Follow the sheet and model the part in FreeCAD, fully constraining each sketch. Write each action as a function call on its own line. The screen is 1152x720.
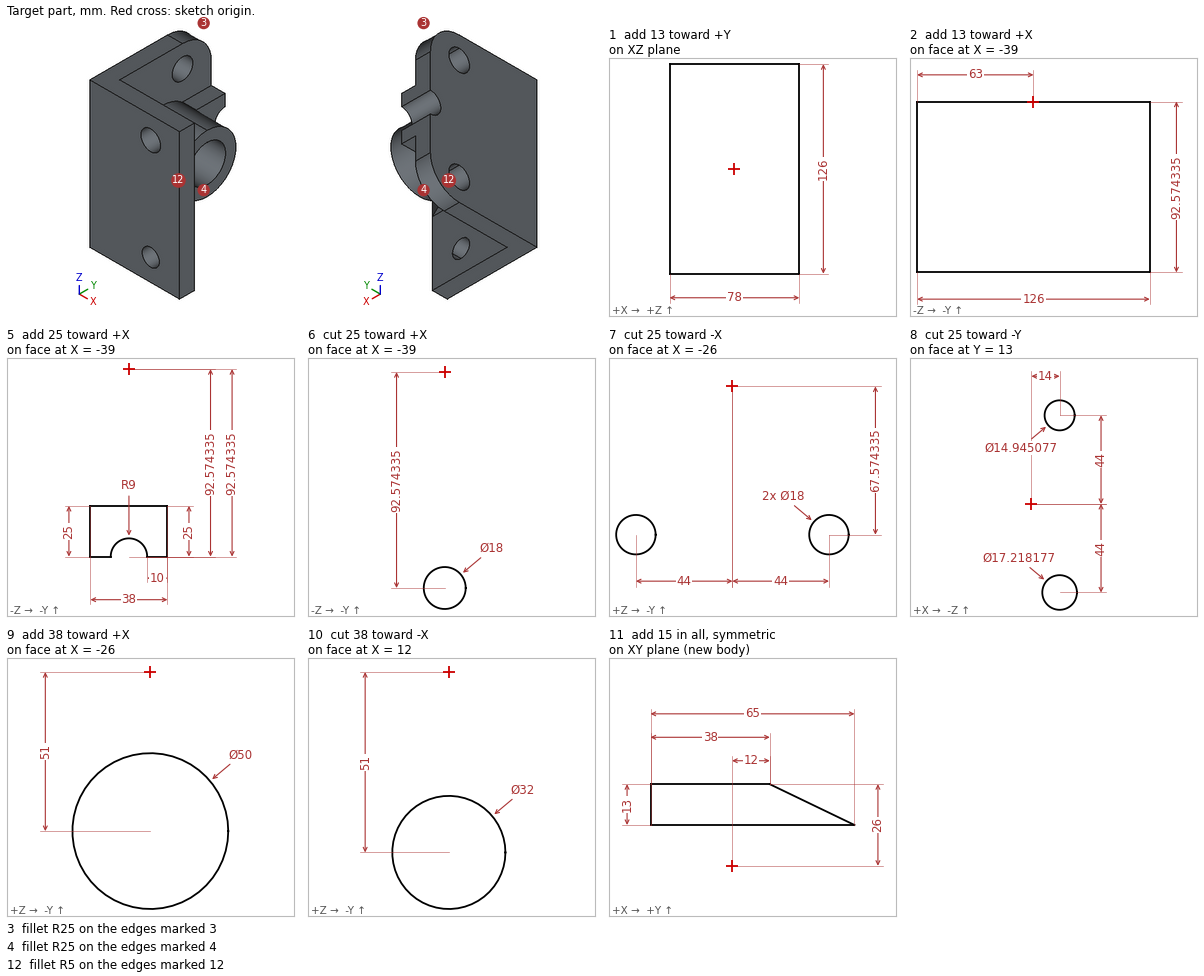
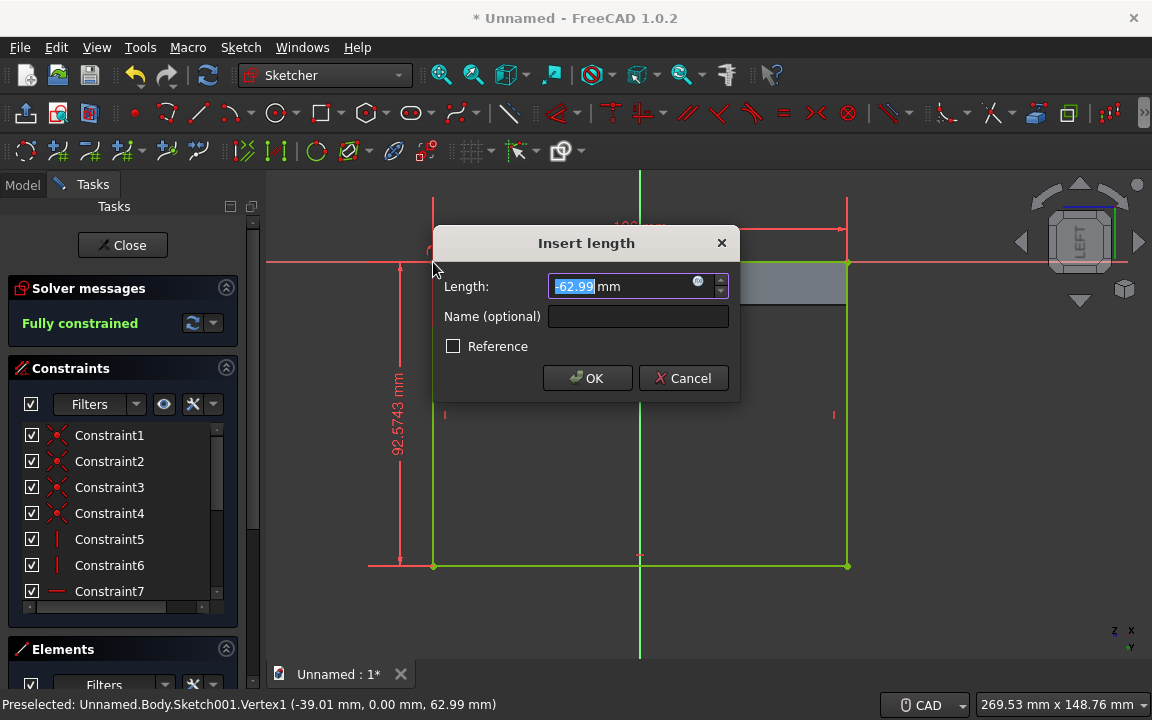
text(-63)
key(Return)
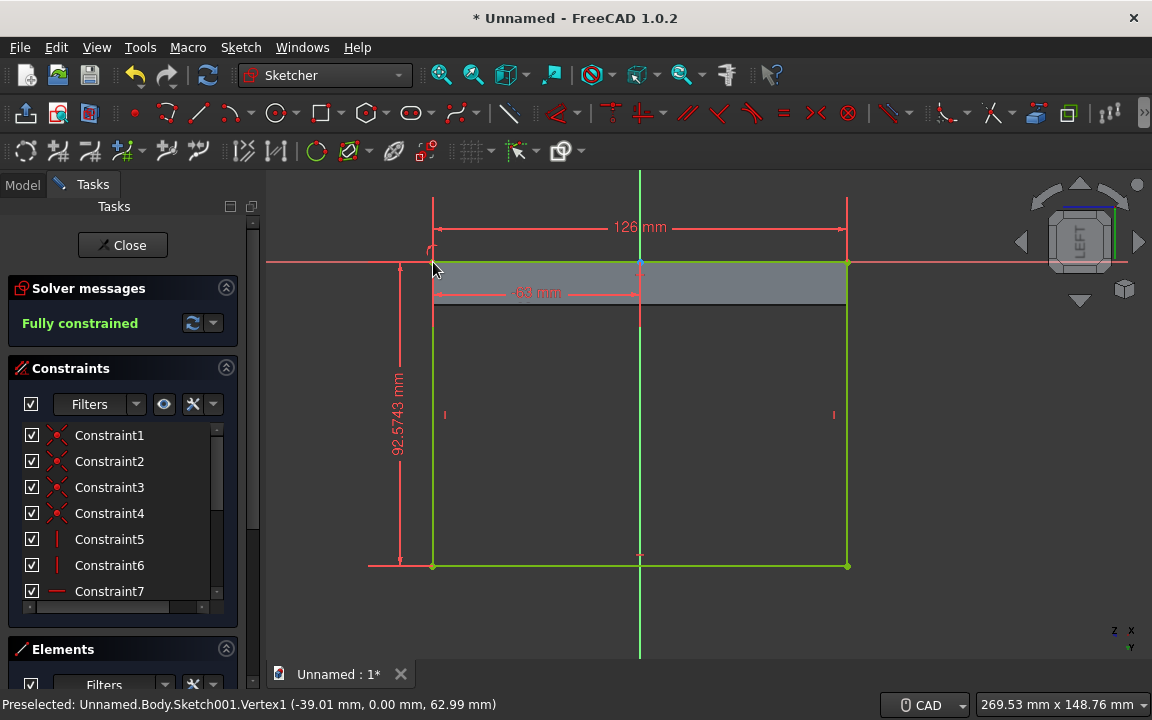
click(123, 245)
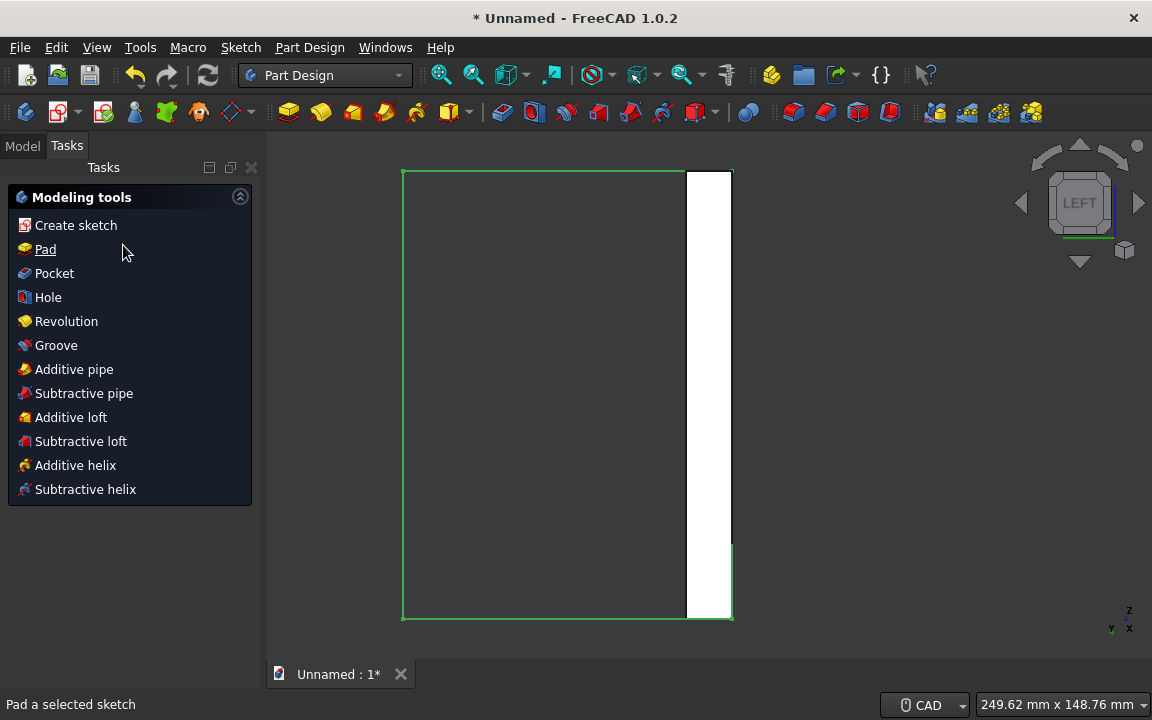
click(290, 112)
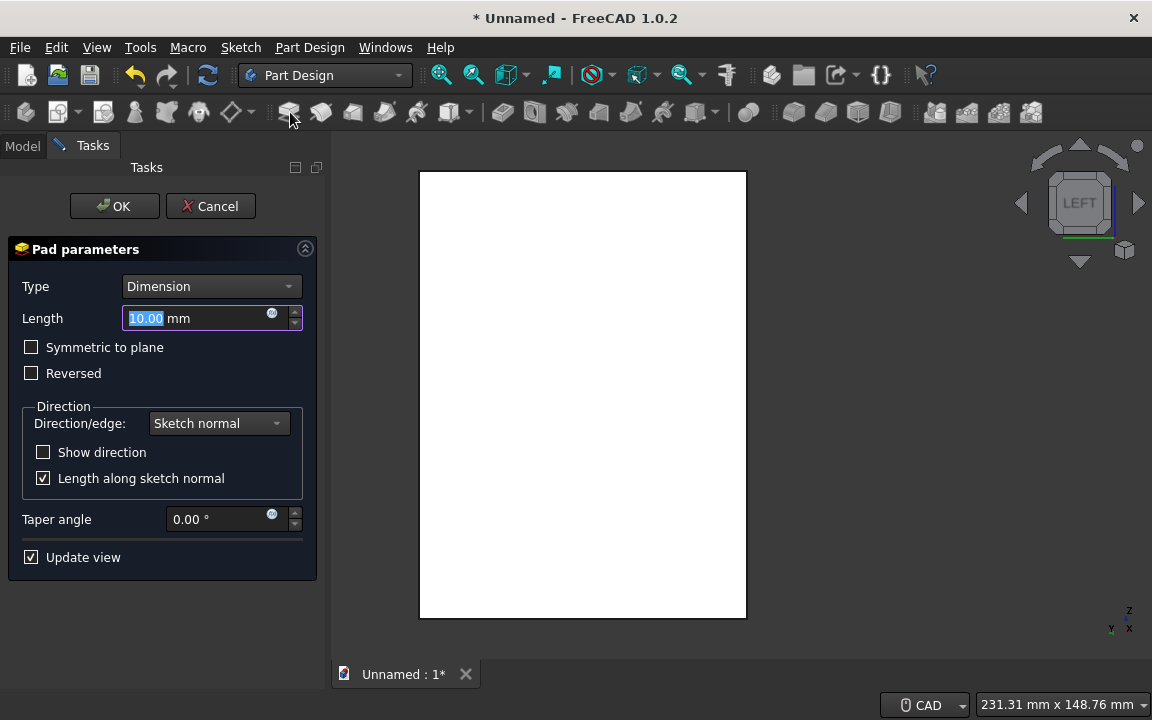
text(13)
key(Tab)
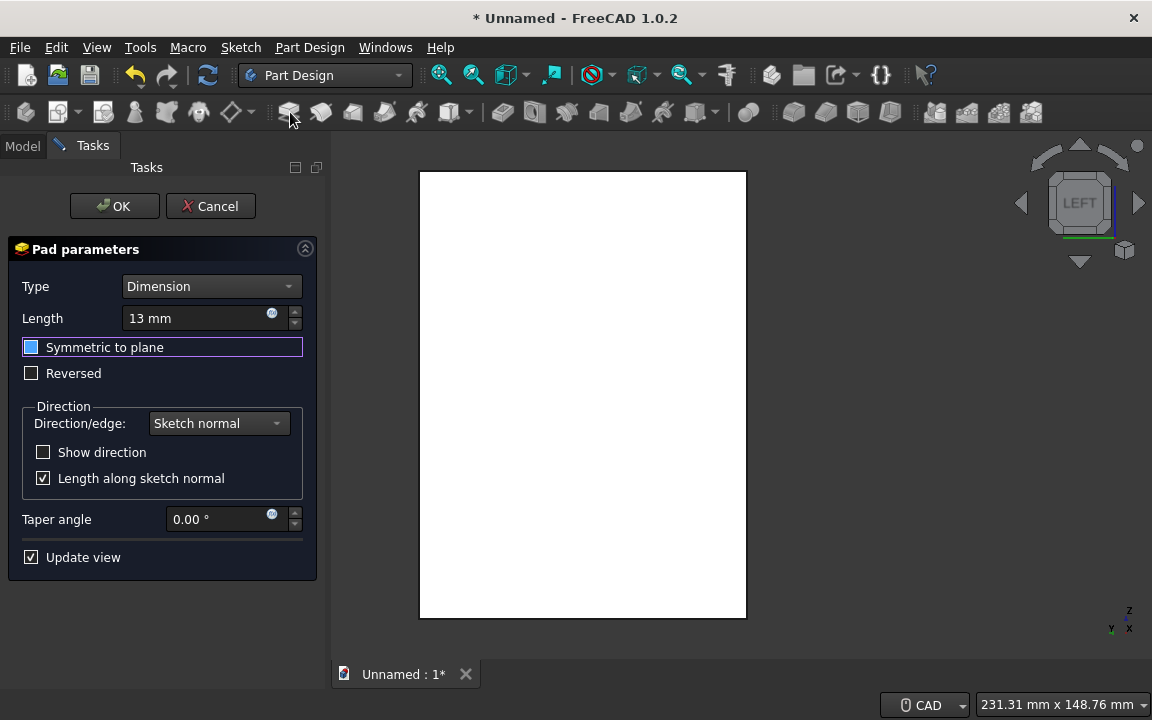
click(30, 373)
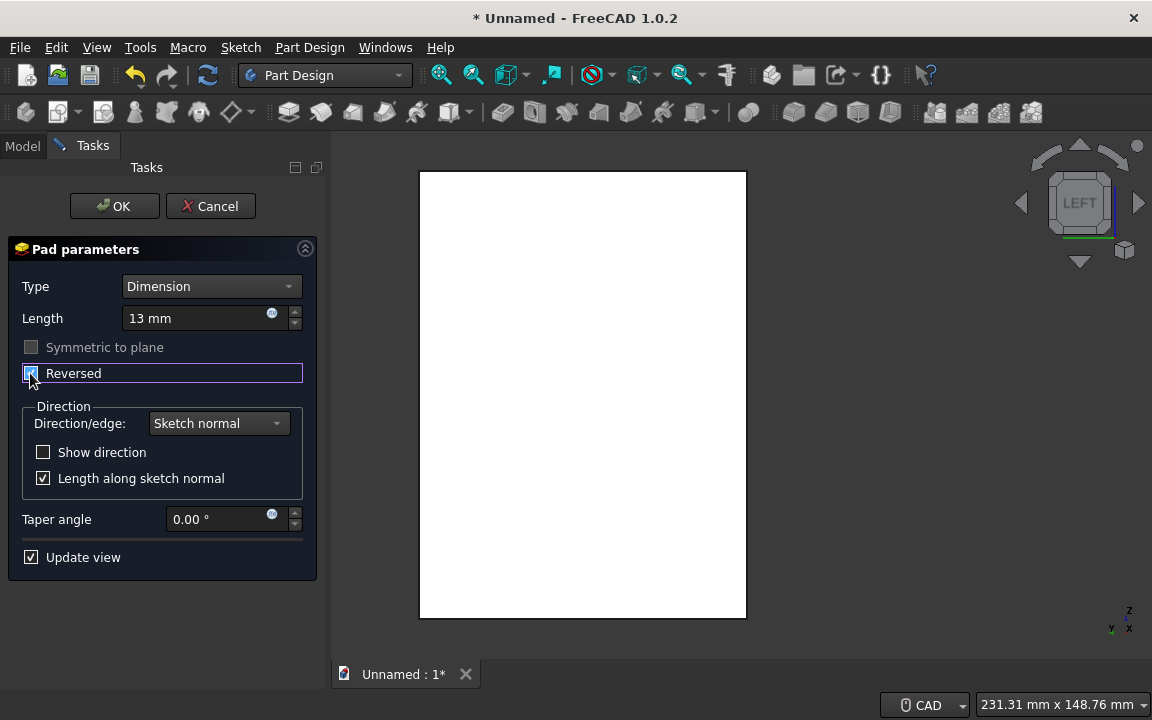
click(115, 206)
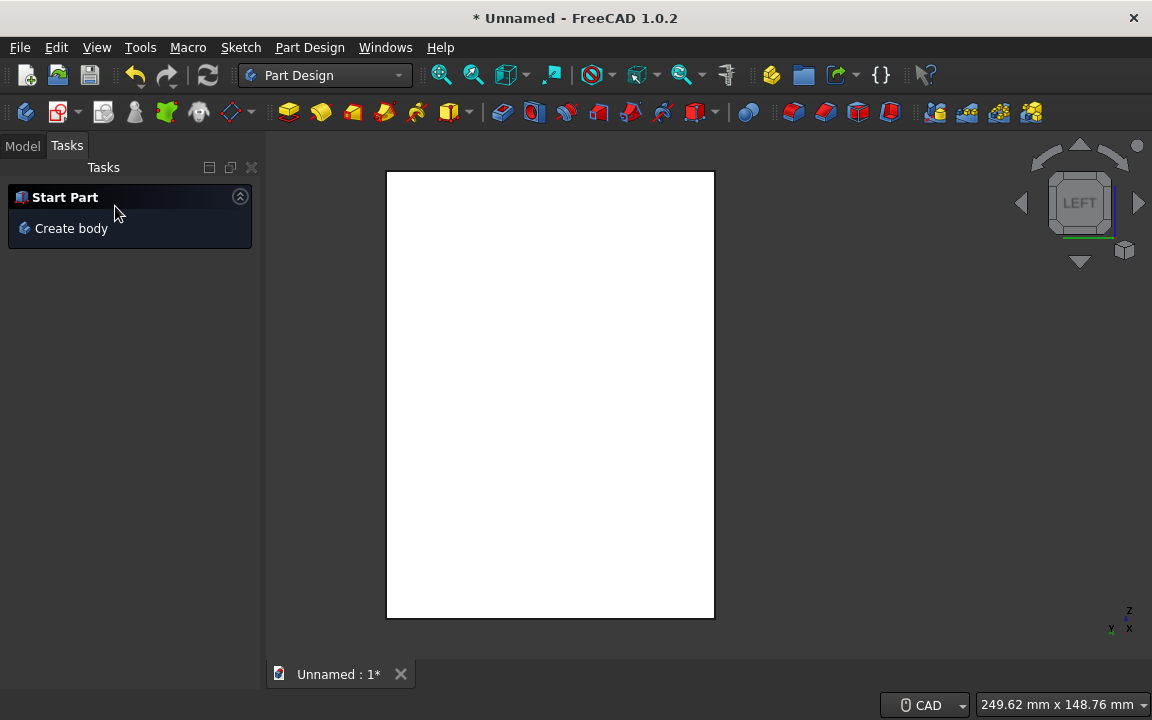
key(0)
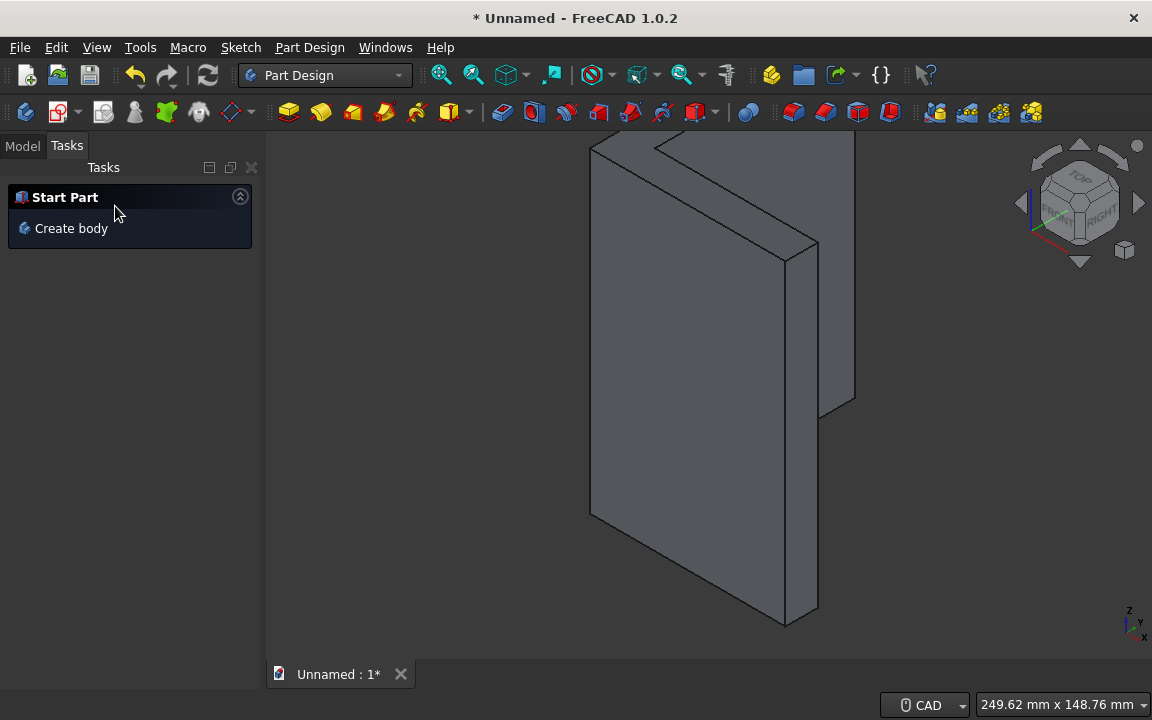
key(v)
key(f)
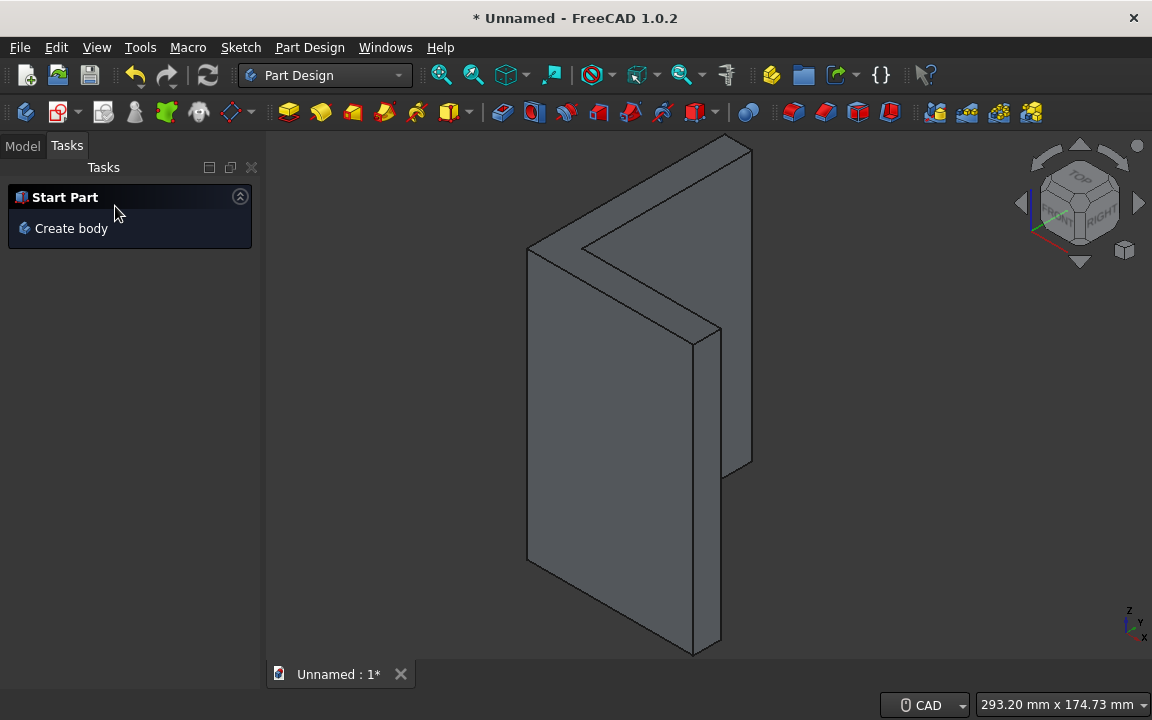
key(2)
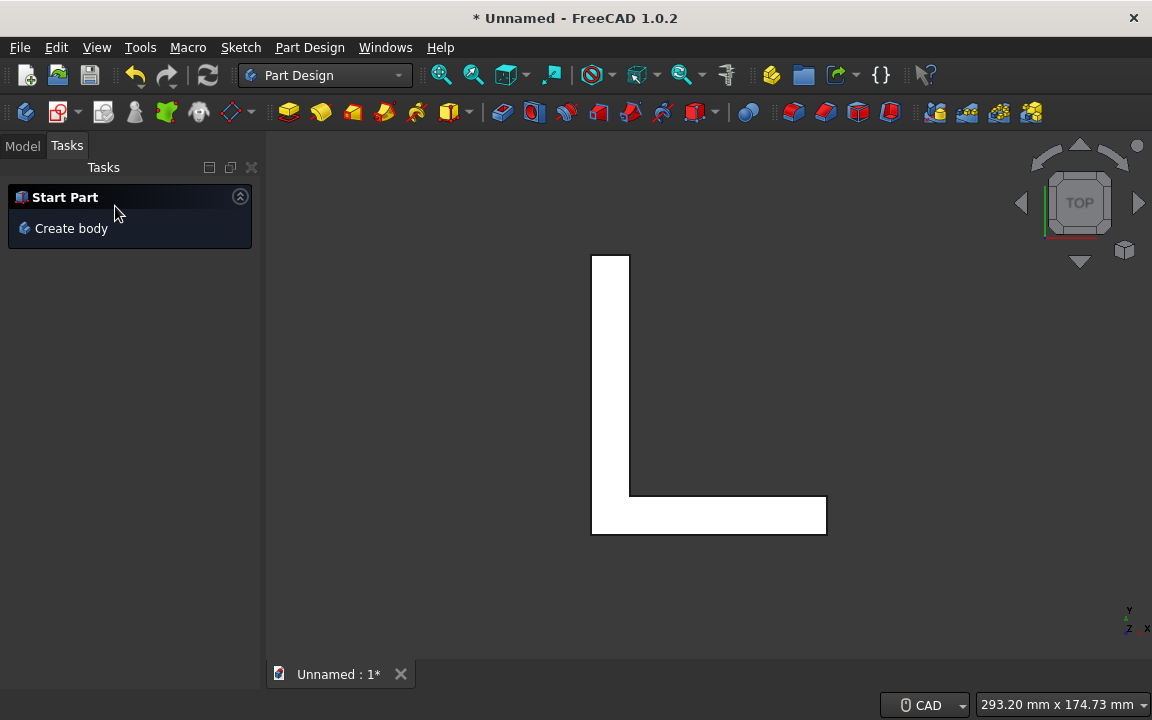
click(611, 254)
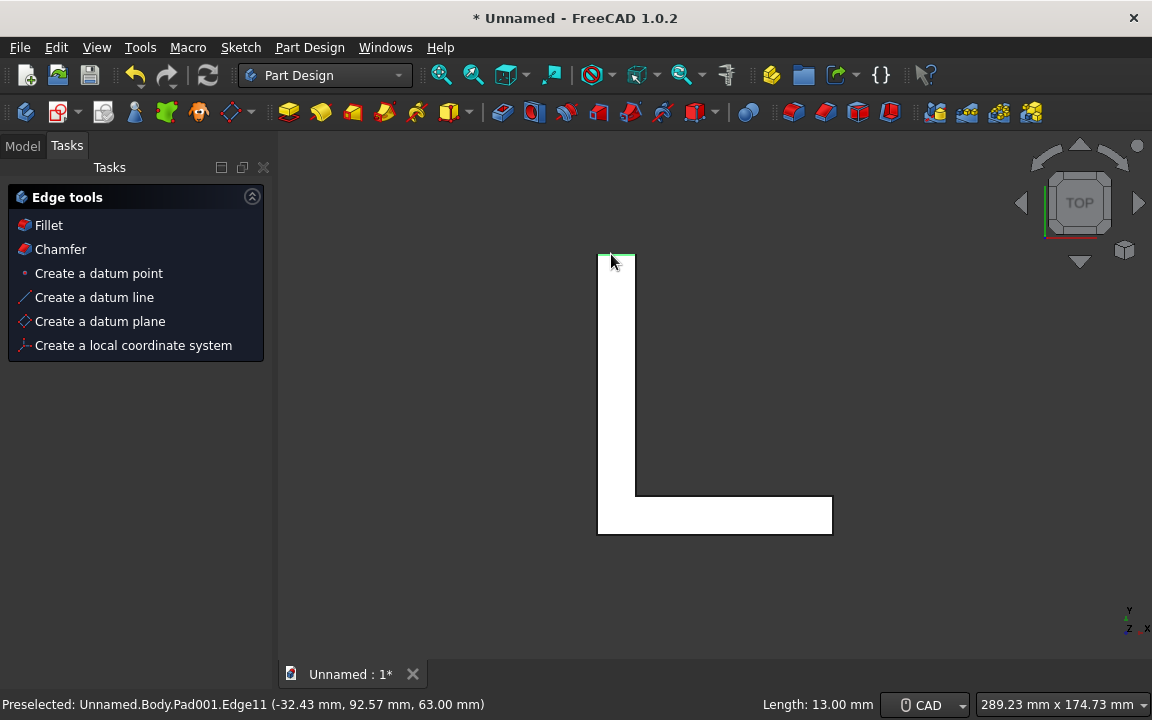
click(794, 112)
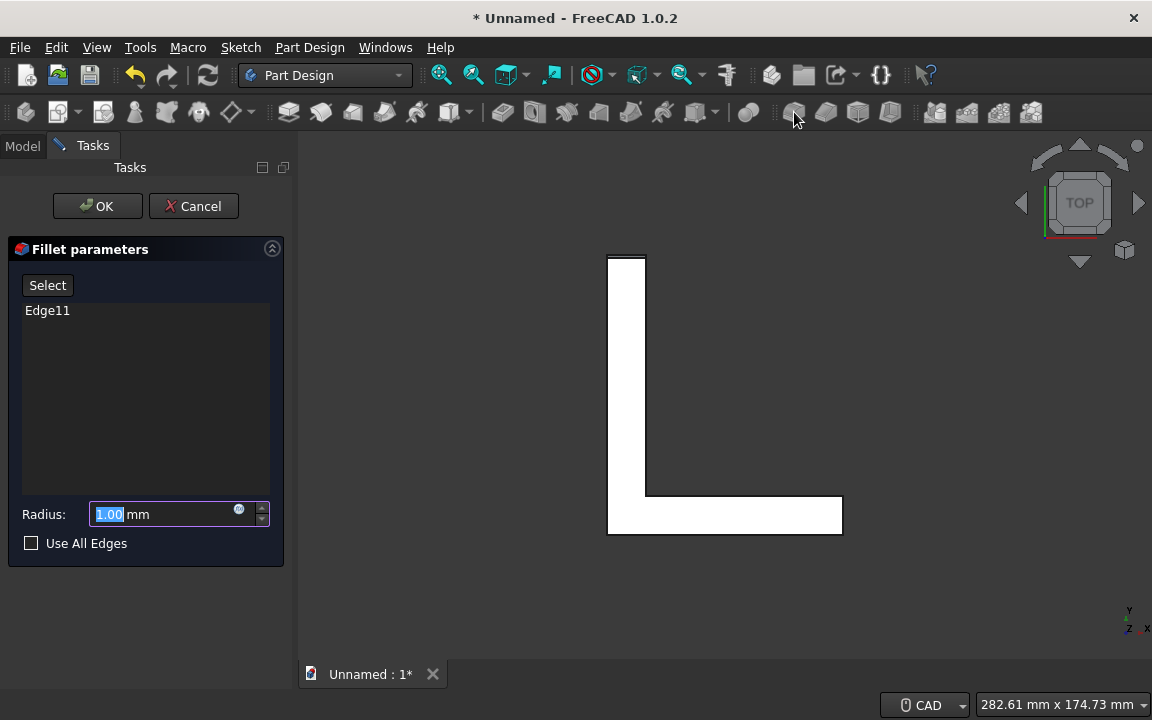
text(25)
key(Tab)